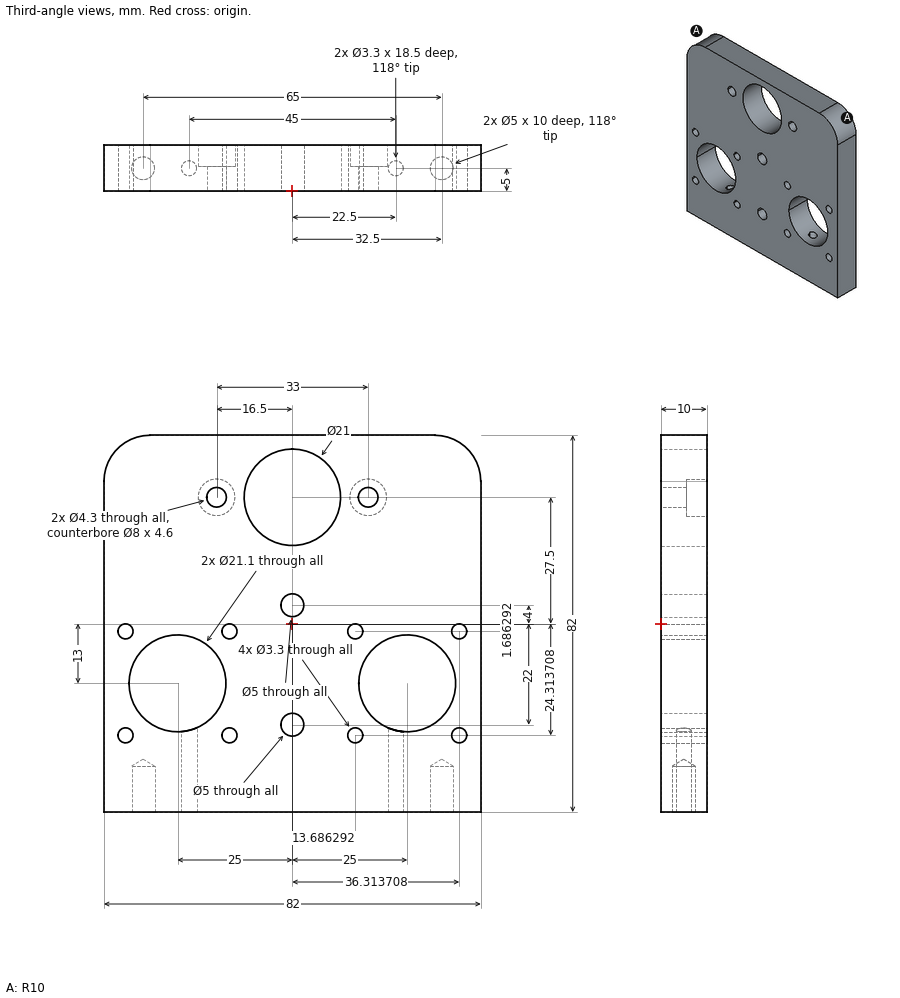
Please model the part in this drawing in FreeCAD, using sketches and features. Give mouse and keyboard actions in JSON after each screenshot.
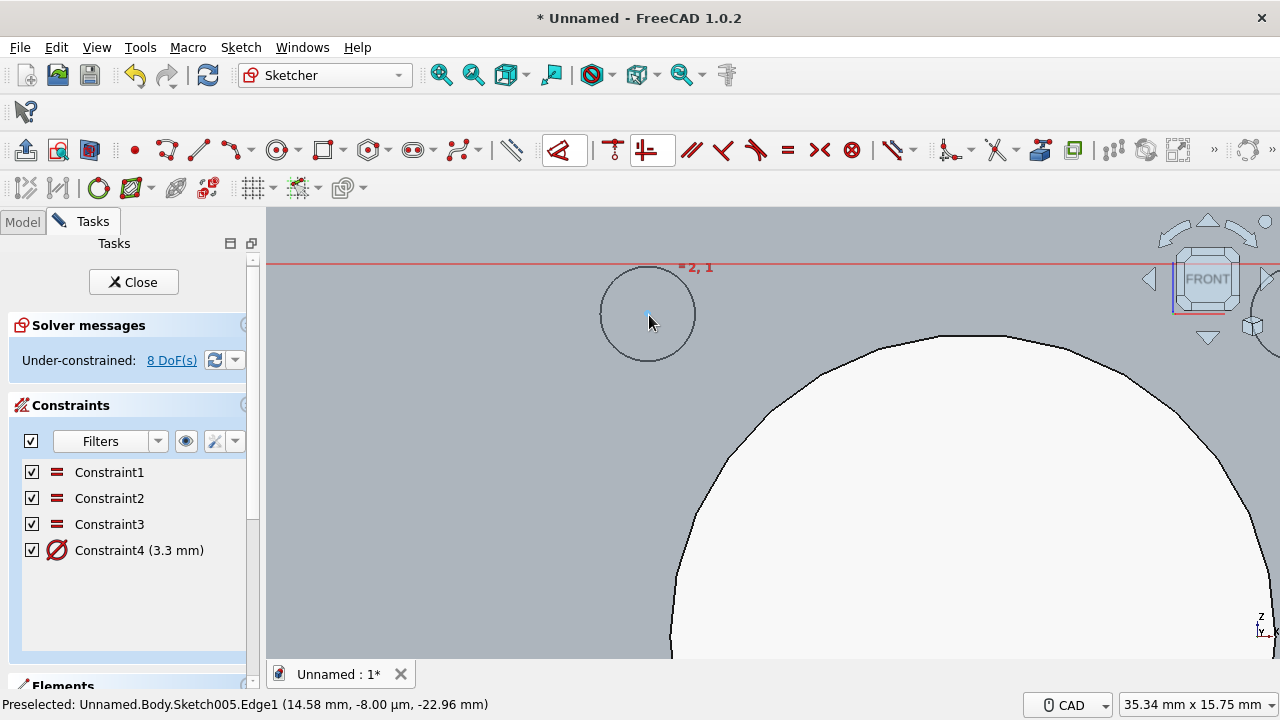
{"action": "left_click", "coordinate": [648, 314]}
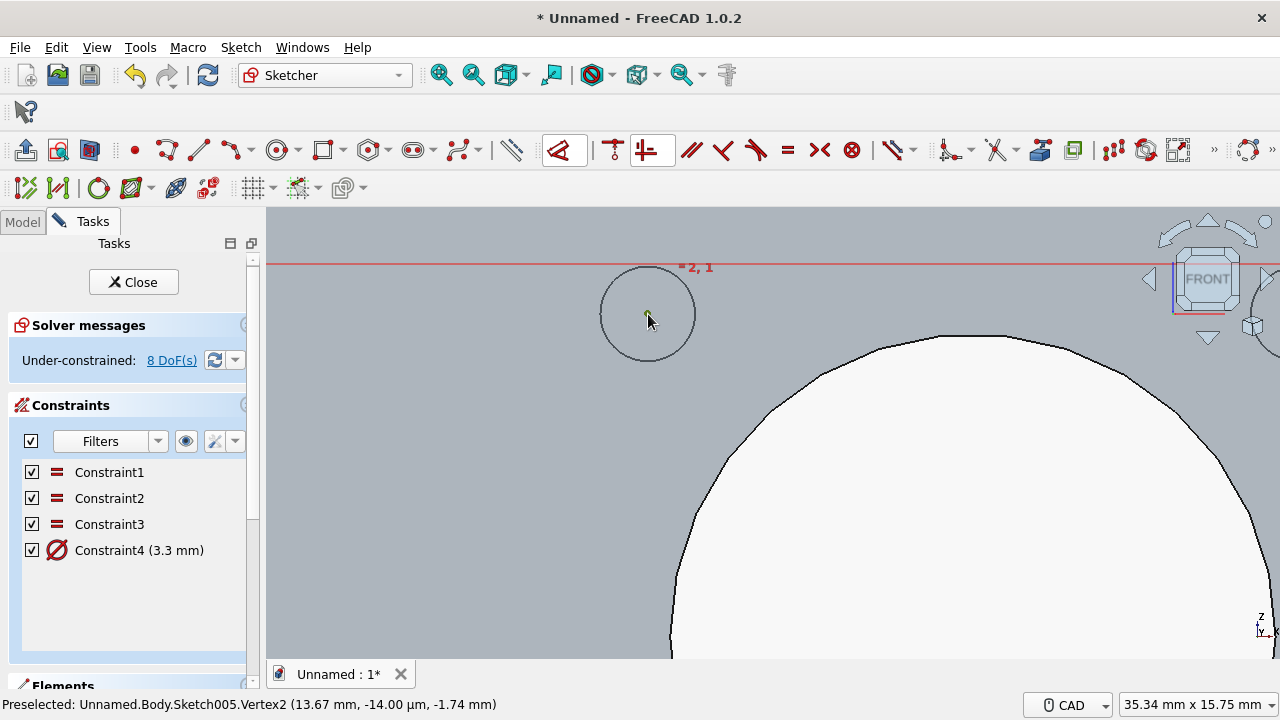
{"action": "left_click", "coordinate": [582, 150]}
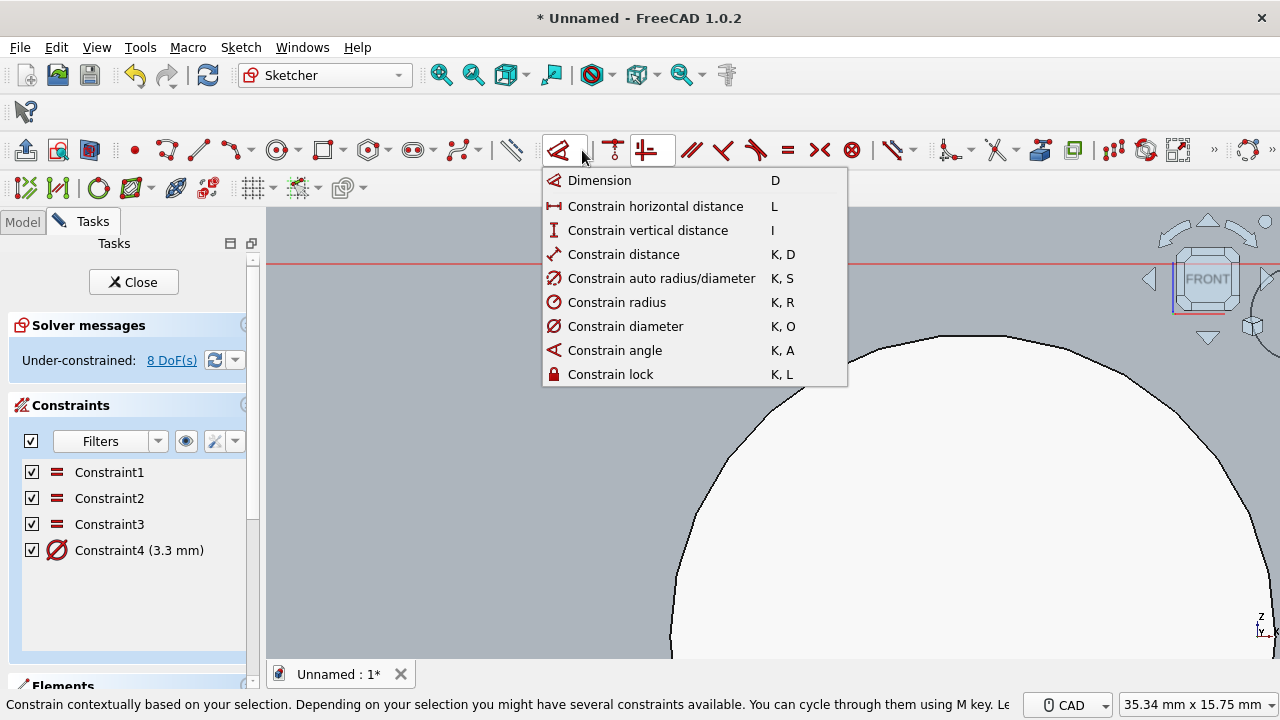
{"action": "left_click", "coordinate": [695, 230]}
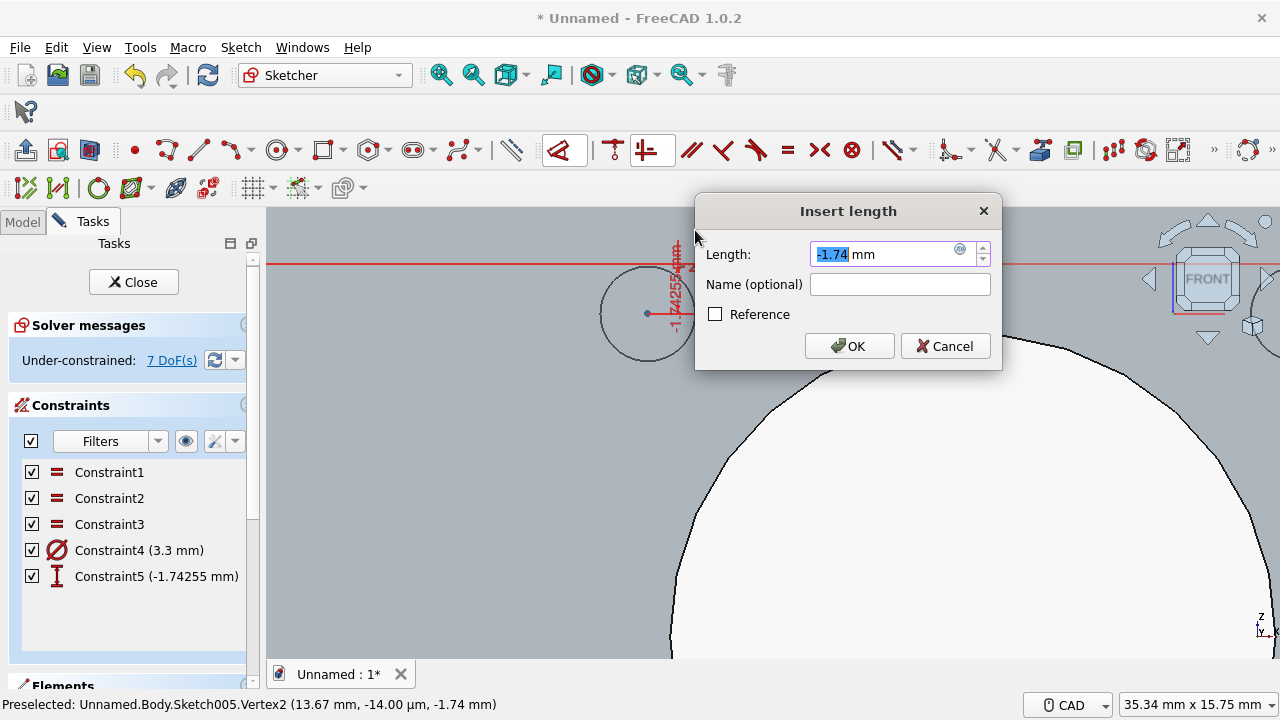
{"action": "type", "text": "-1.686292"}
{"action": "key", "text": "Return"}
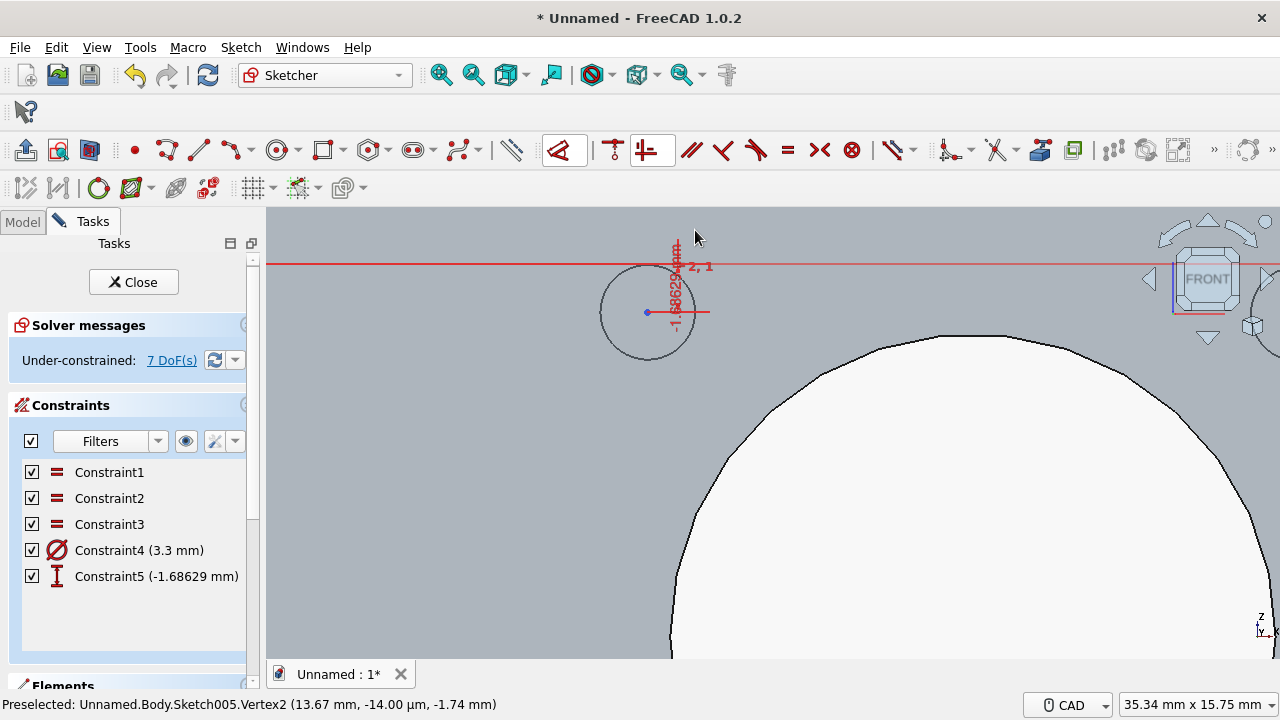
{"action": "scroll", "coordinate": [649, 315], "scroll_direction": "down", "scroll_amount": 5}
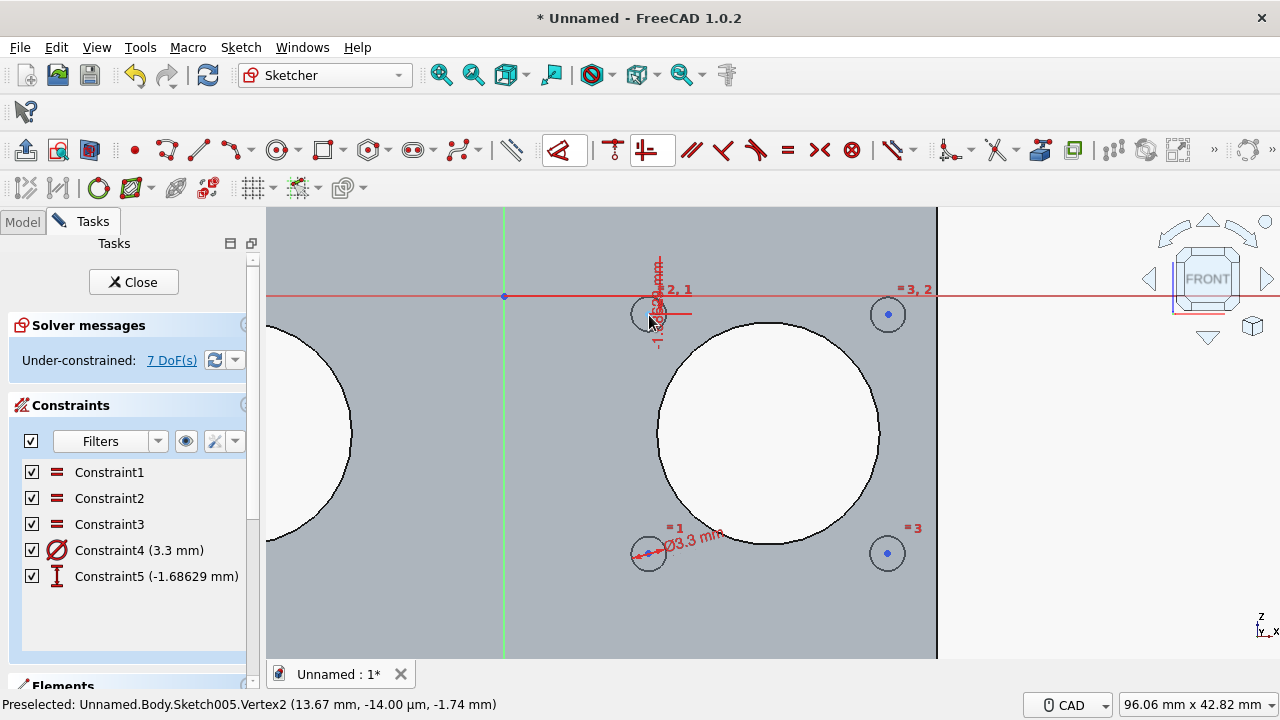
{"action": "scroll", "coordinate": [888, 315], "scroll_direction": "up", "scroll_amount": 5}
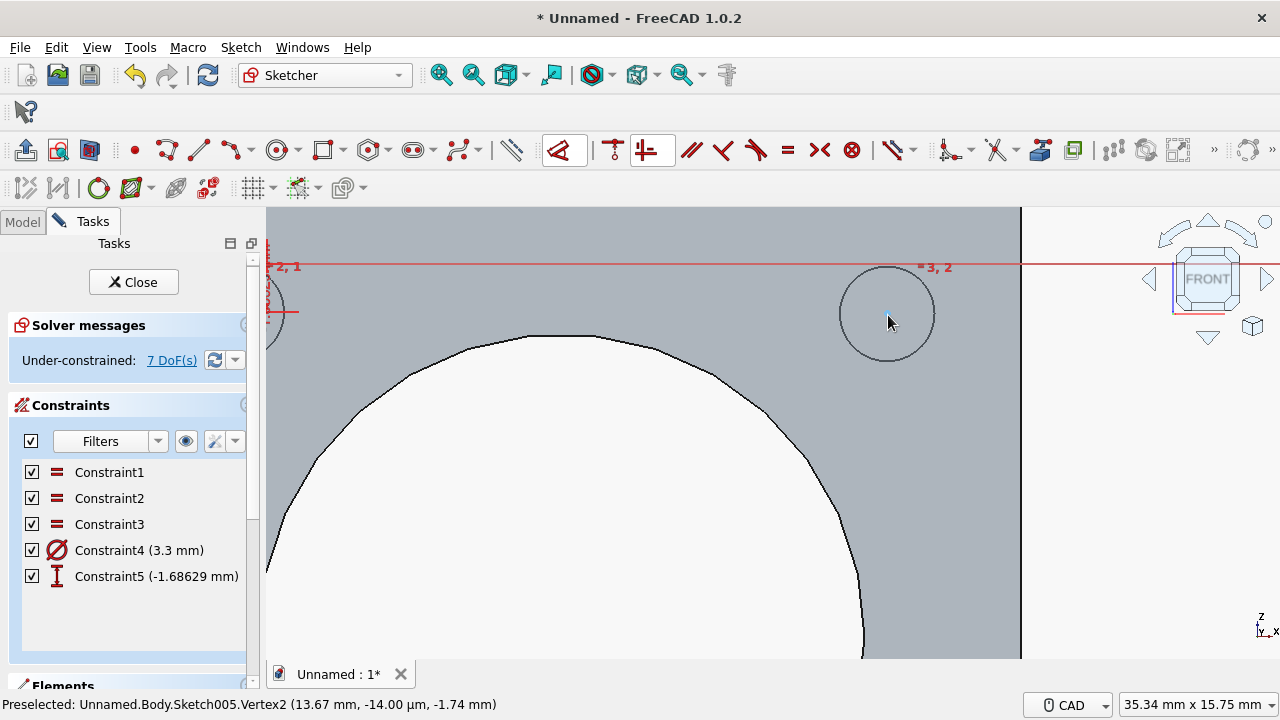
{"action": "left_click", "coordinate": [887, 314]}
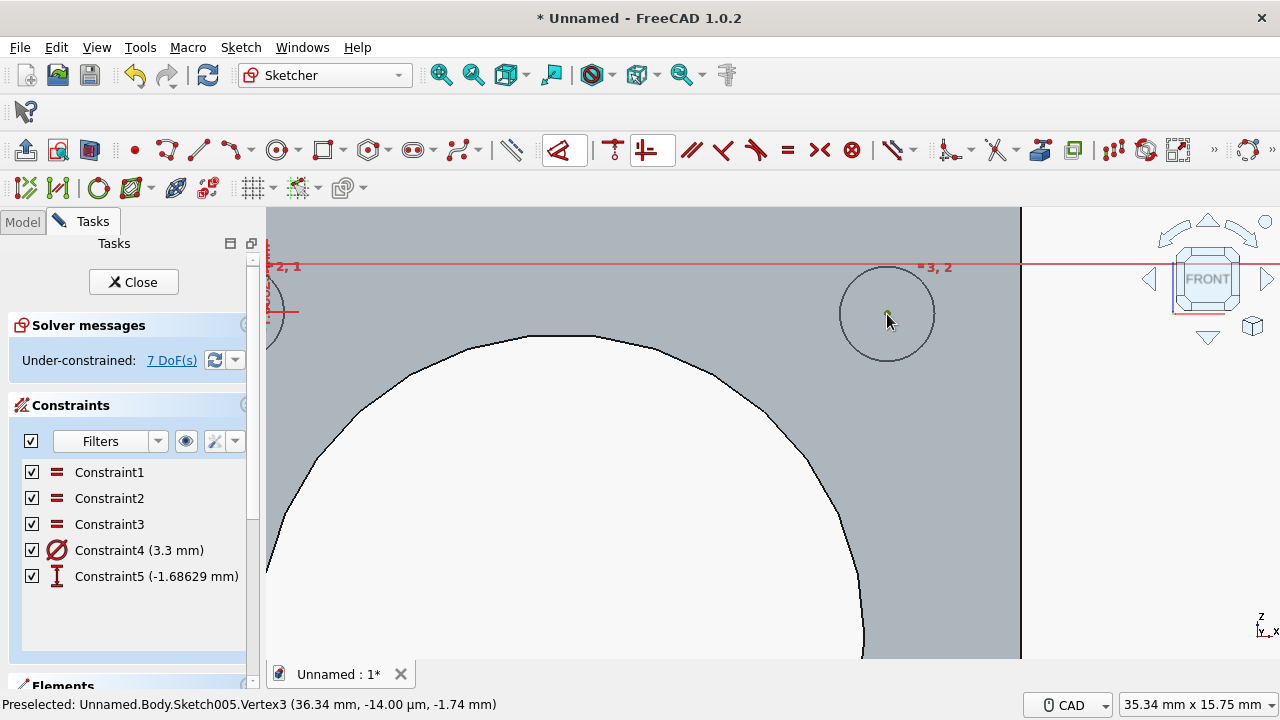
{"action": "key", "text": "i"}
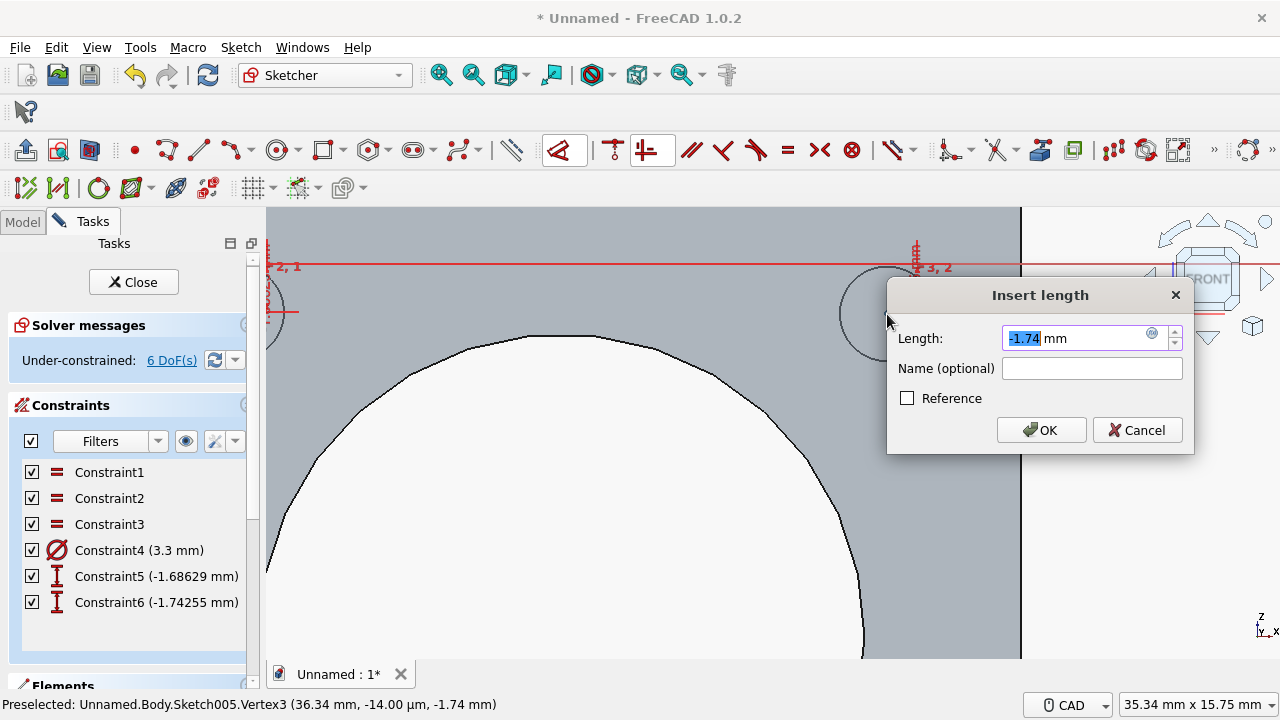
{"action": "type", "text": "-1.686292"}
{"action": "key", "text": "Return"}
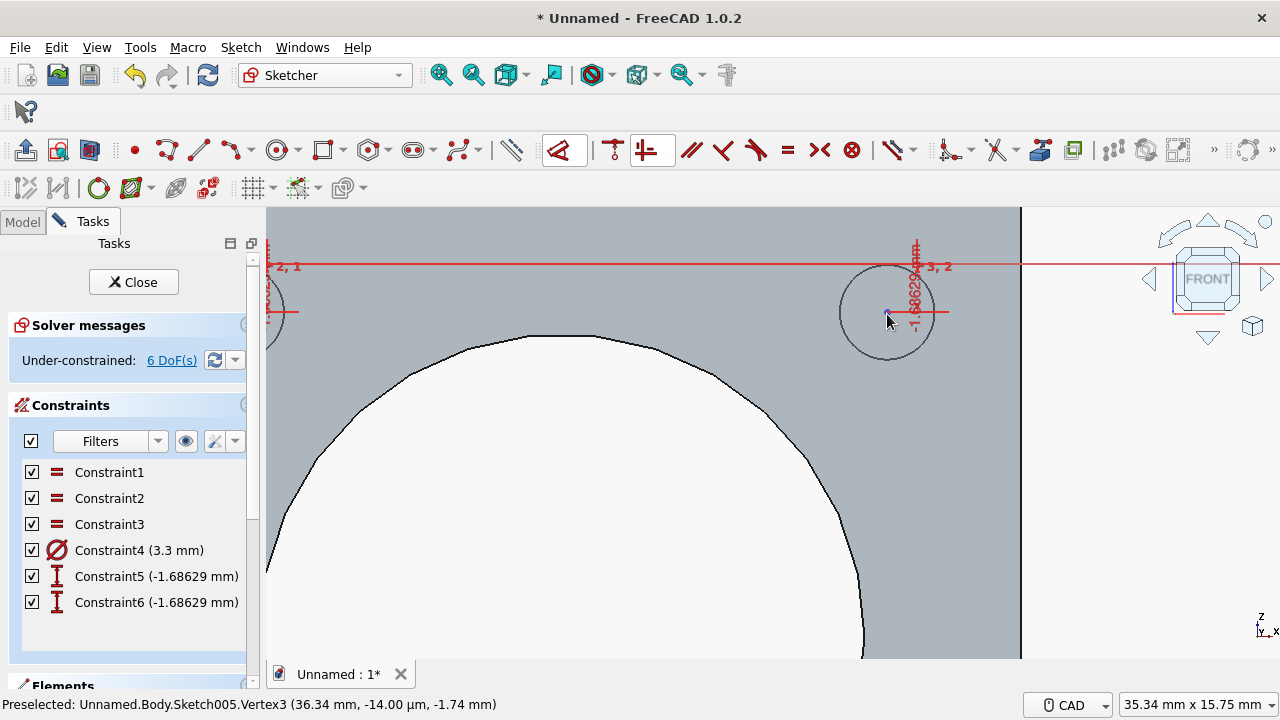
{"action": "scroll", "coordinate": [888, 315], "scroll_direction": "down", "scroll_amount": 5}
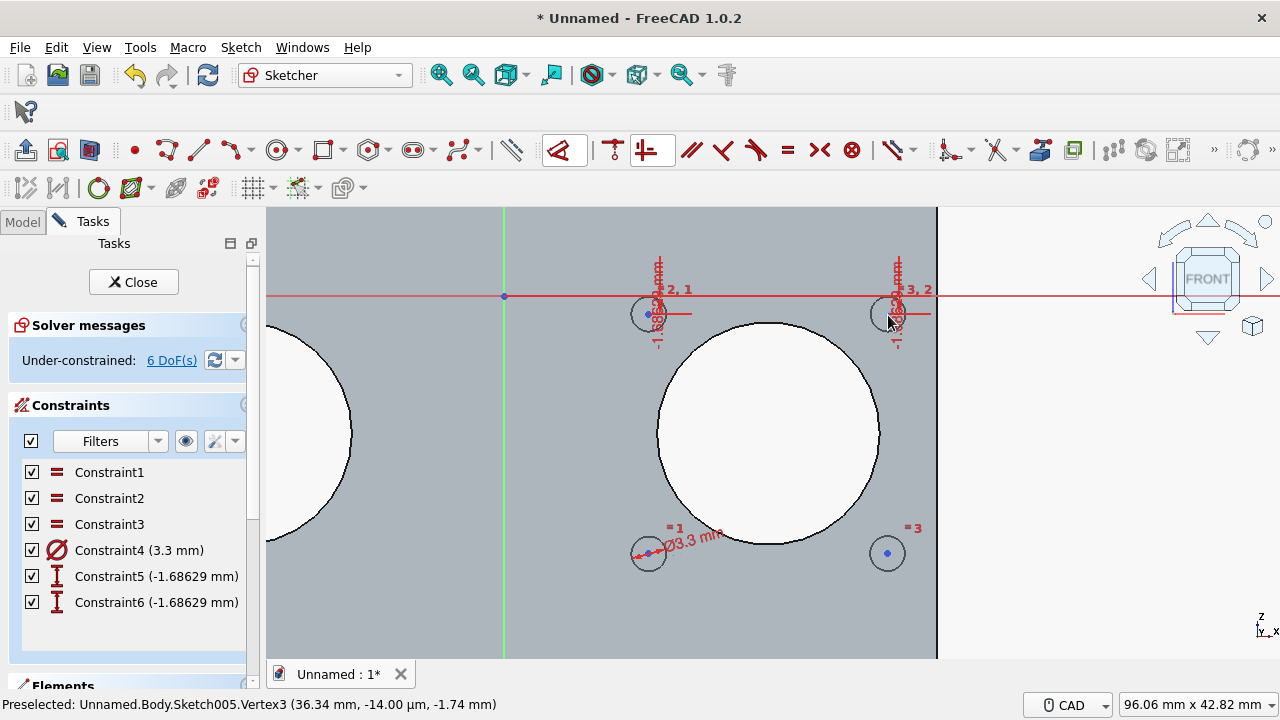
{"action": "left_click", "coordinate": [649, 554]}